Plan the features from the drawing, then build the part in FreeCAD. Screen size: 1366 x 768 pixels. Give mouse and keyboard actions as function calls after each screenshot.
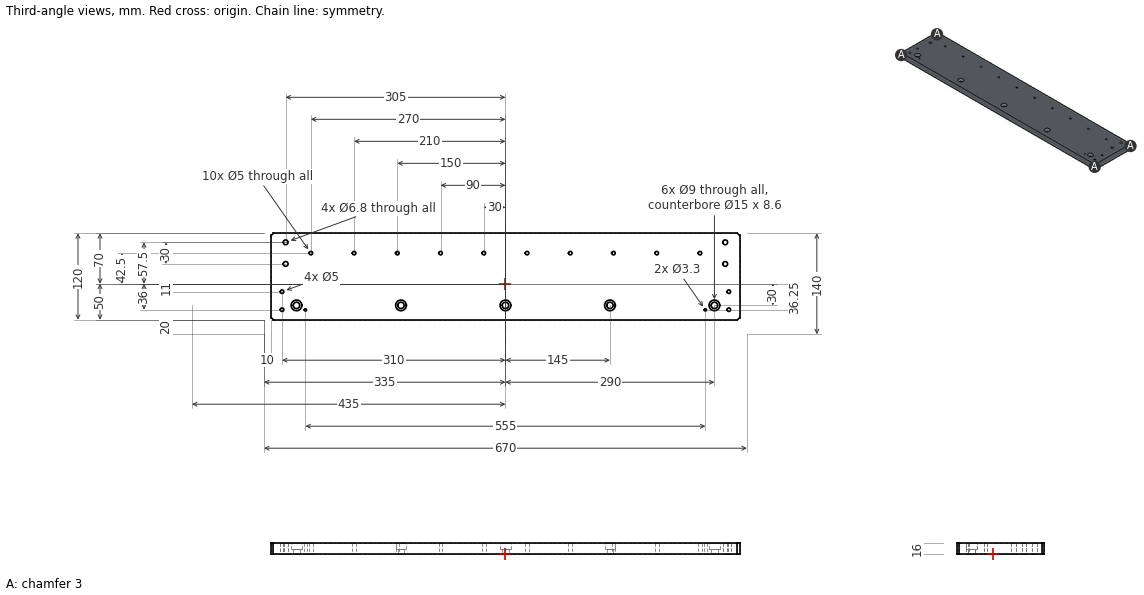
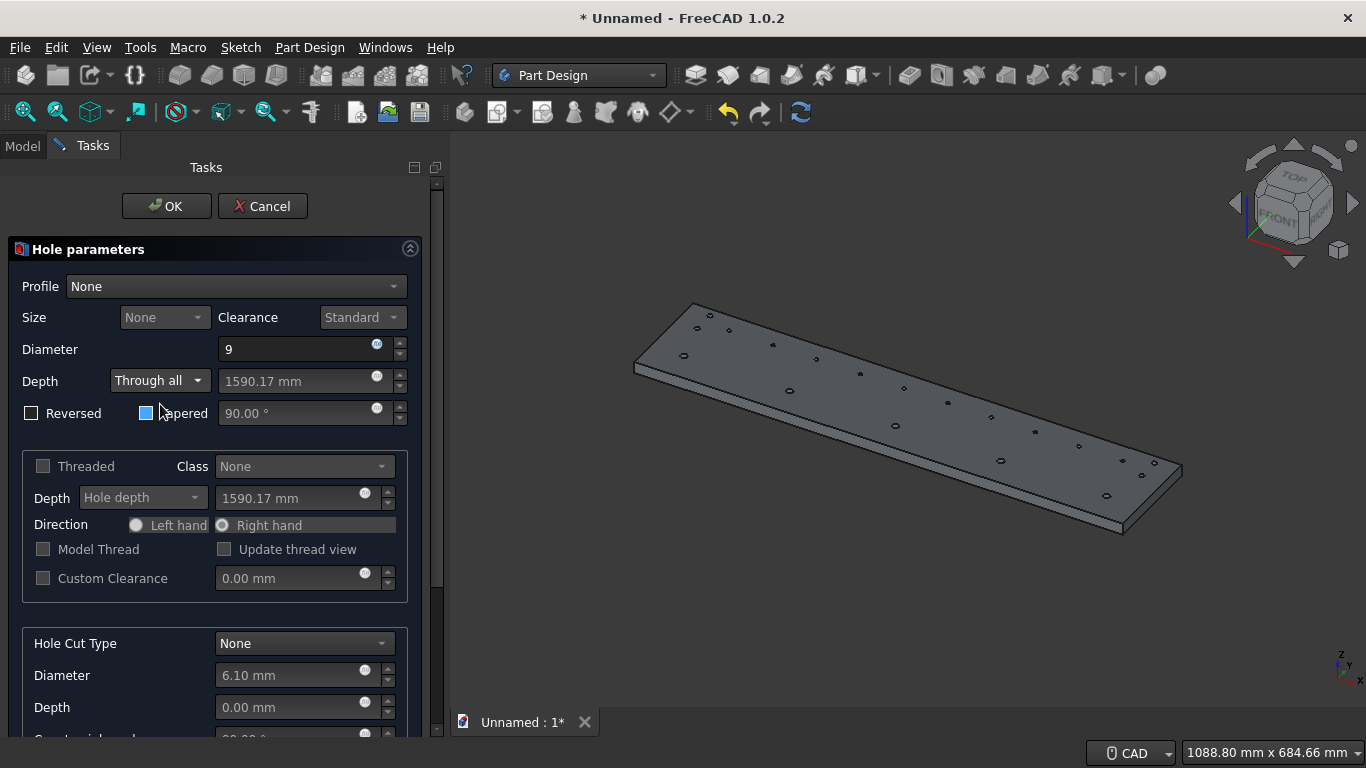
click(306, 644)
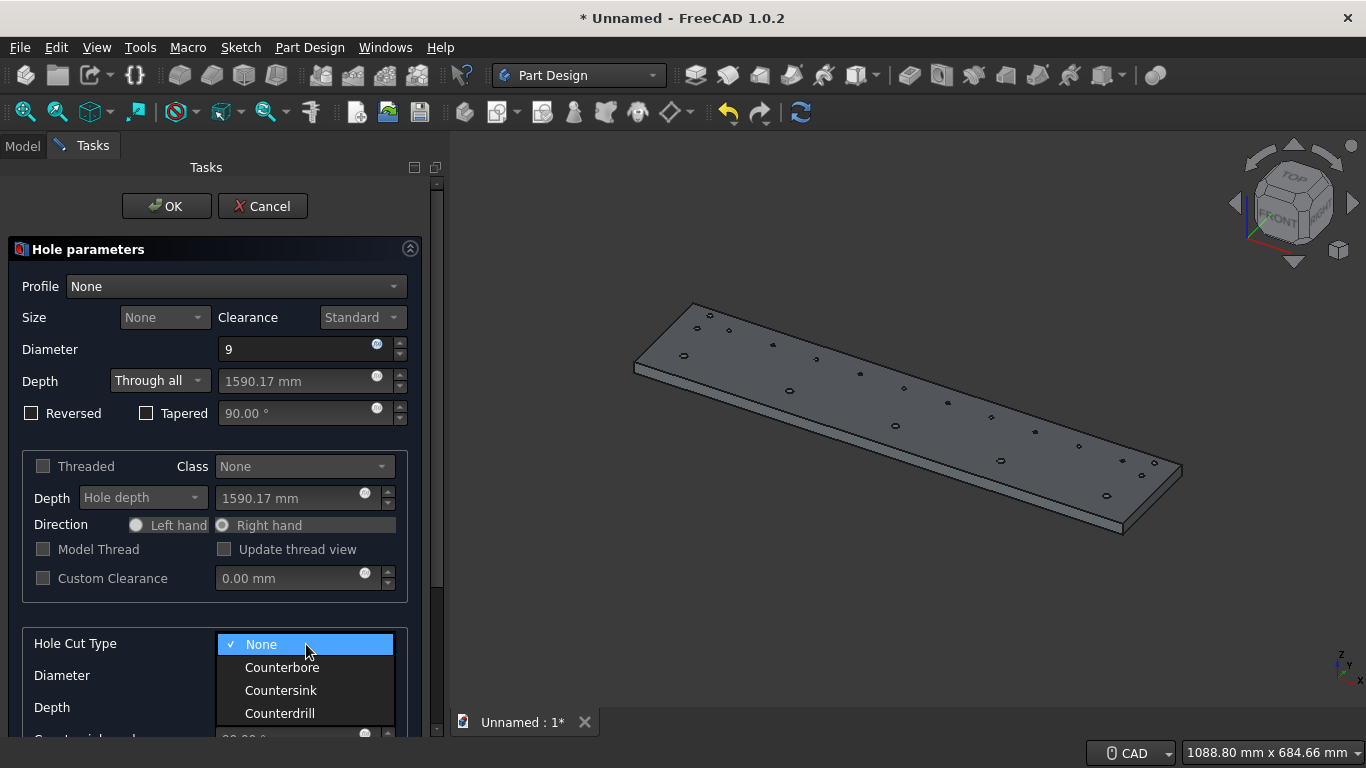
click(304, 668)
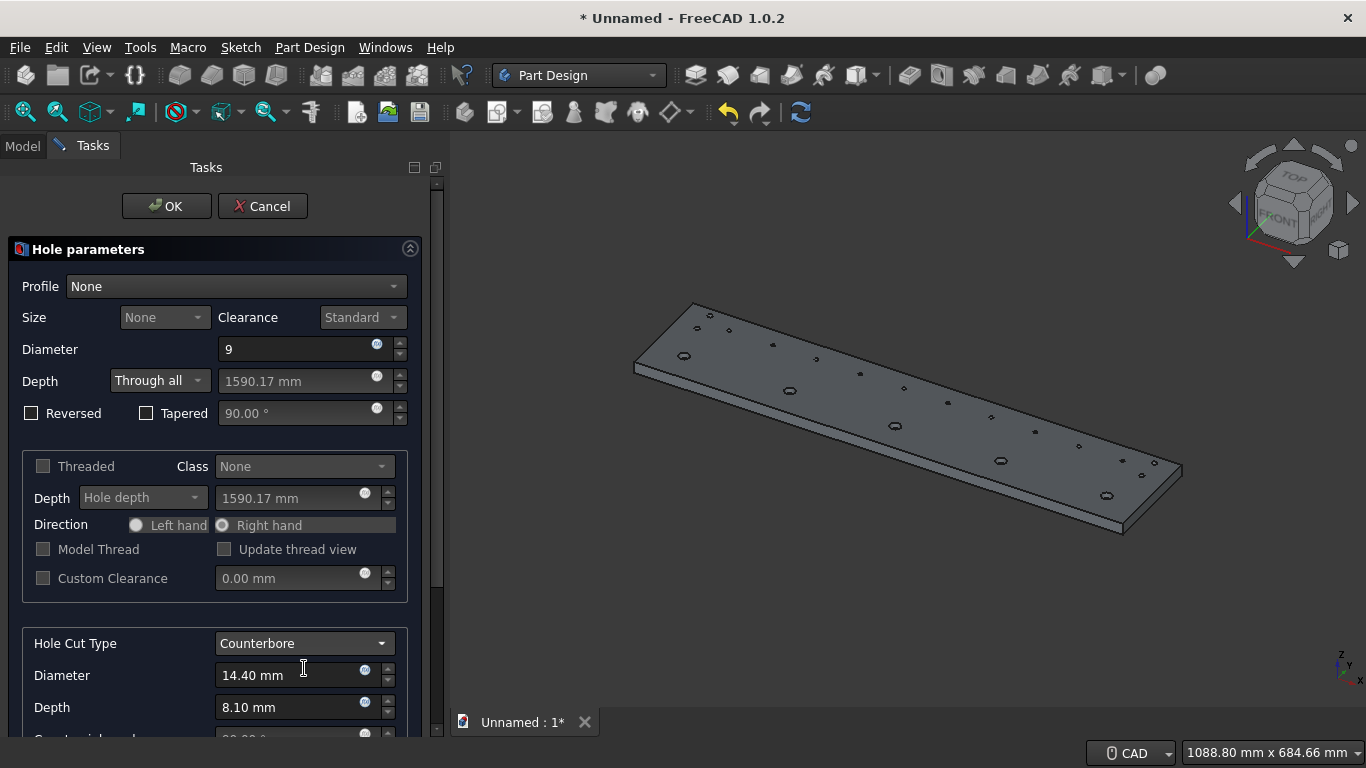
triple_click(298, 675)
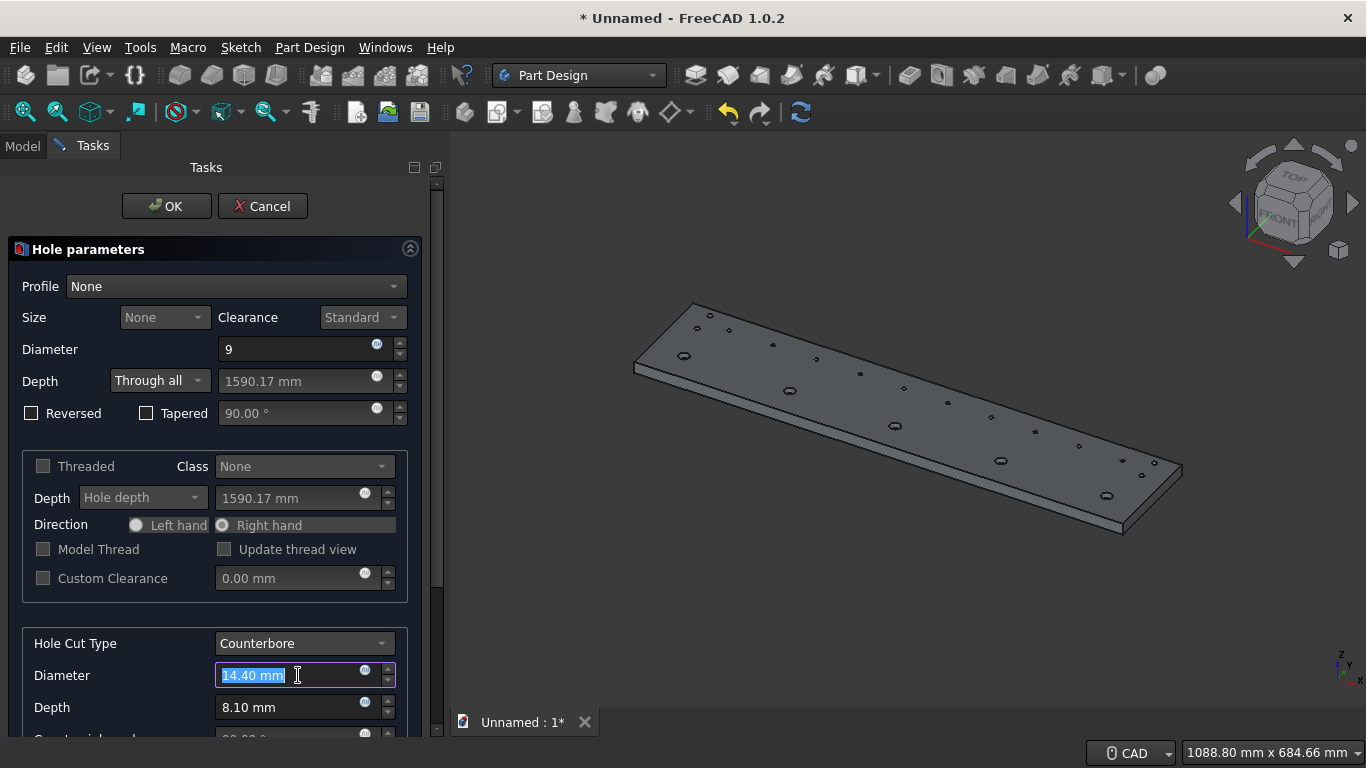
text(15)
key(Tab)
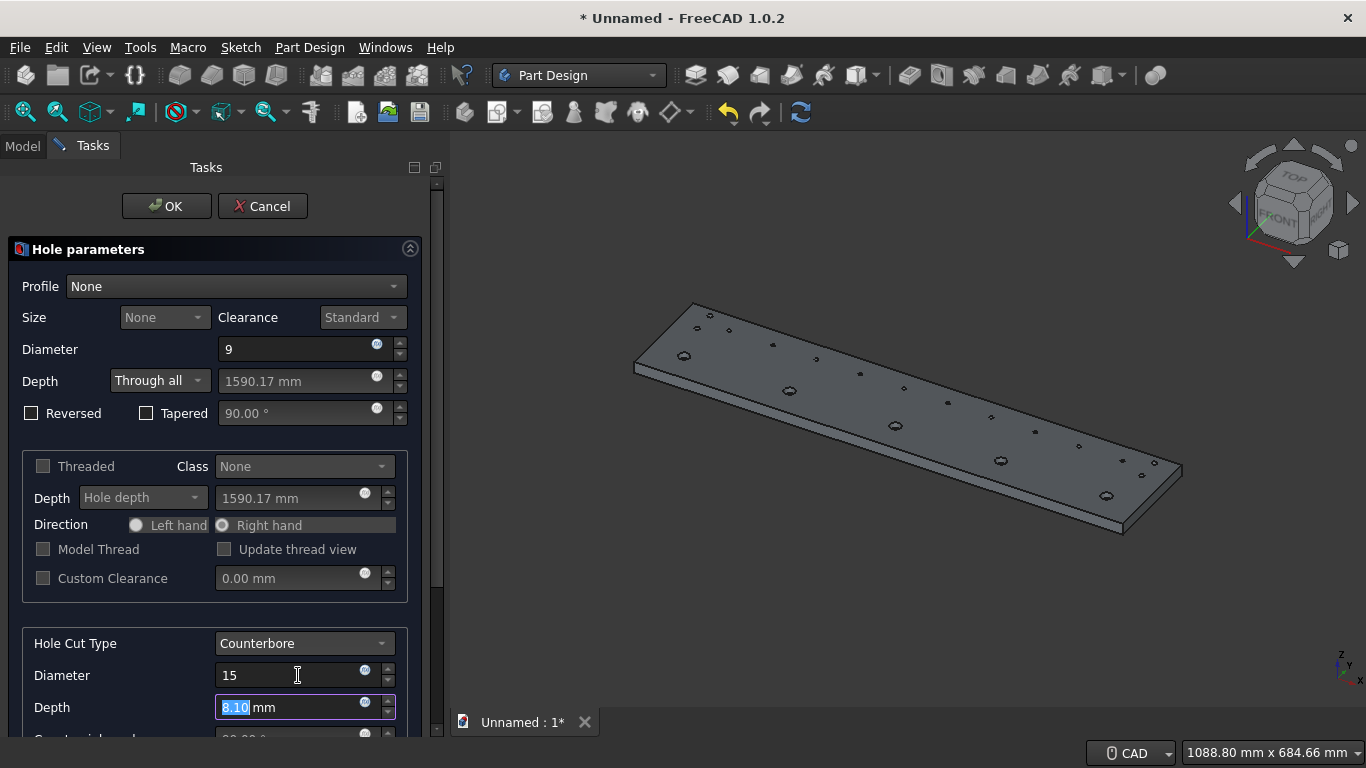
text(8.6)
key(Tab)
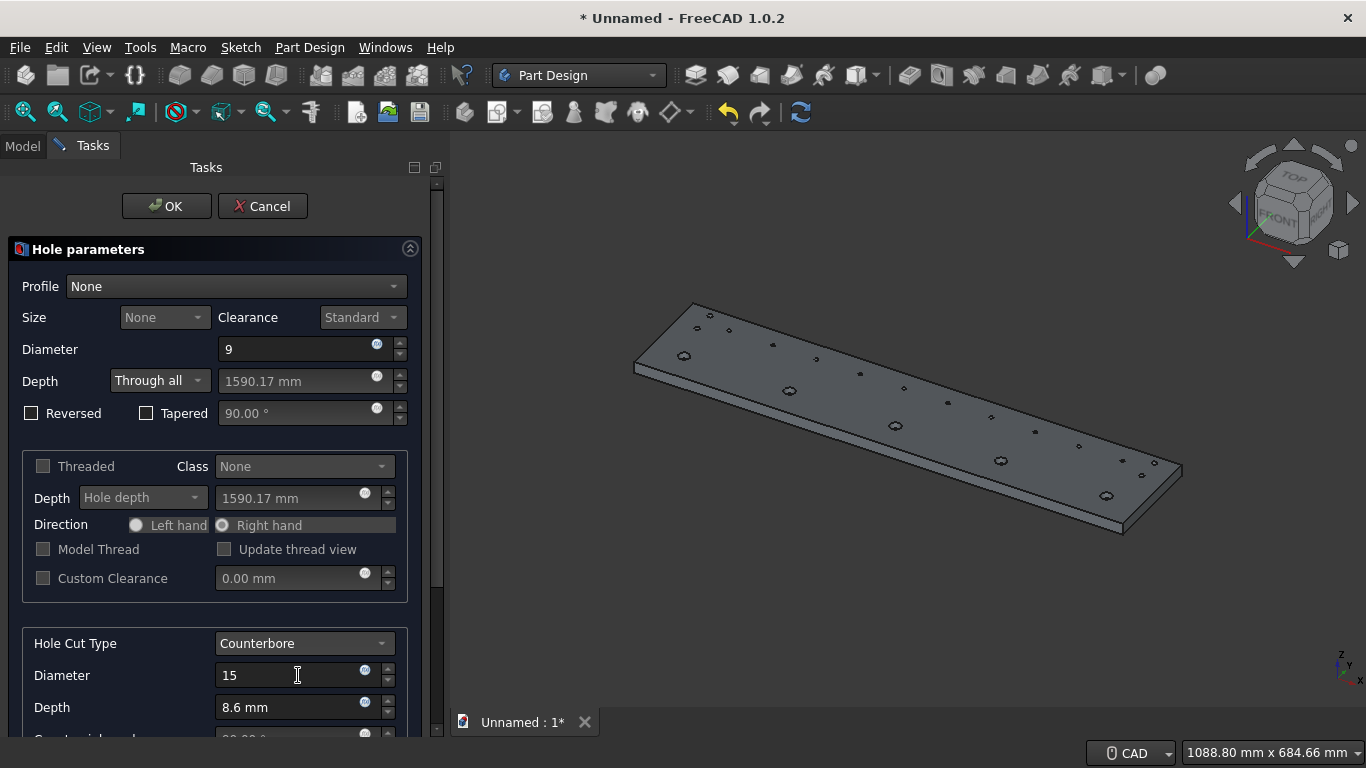
click(167, 206)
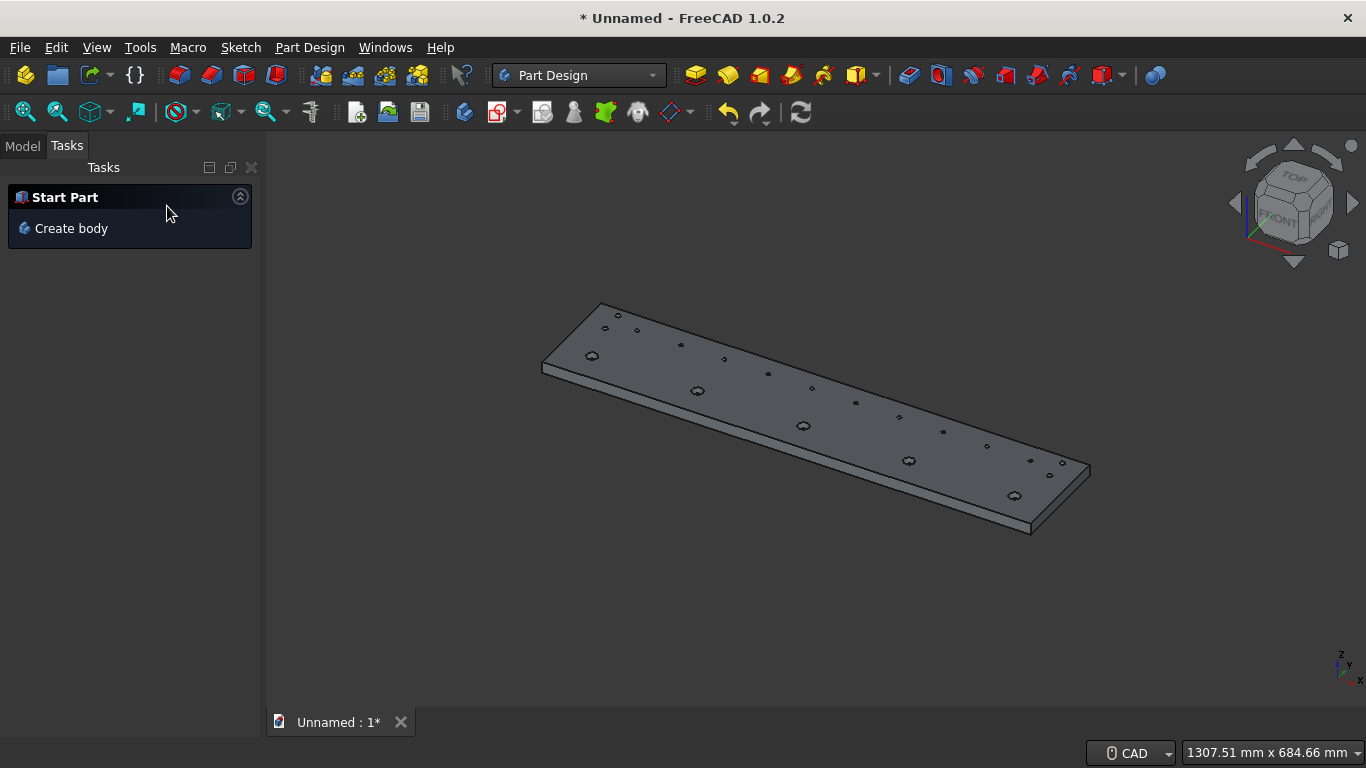
click(677, 366)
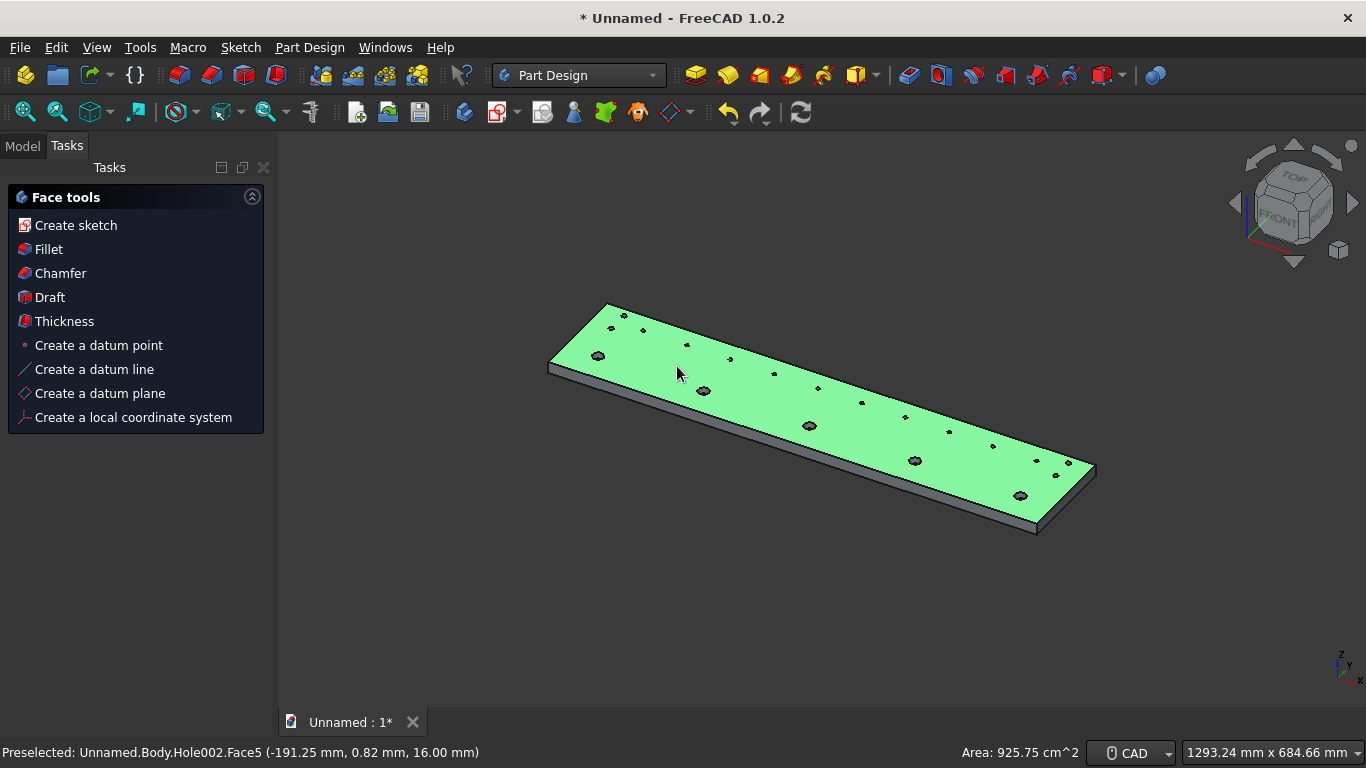
click(498, 112)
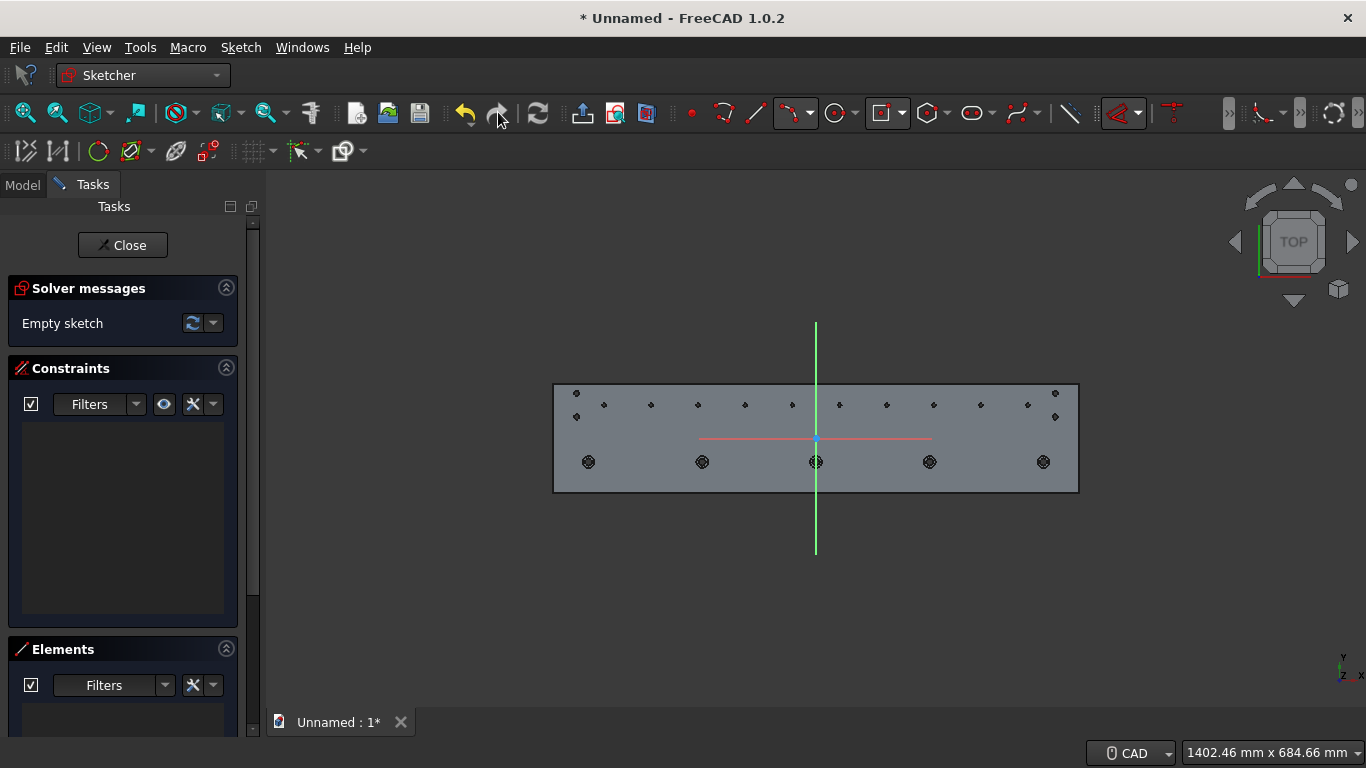
click(904, 114)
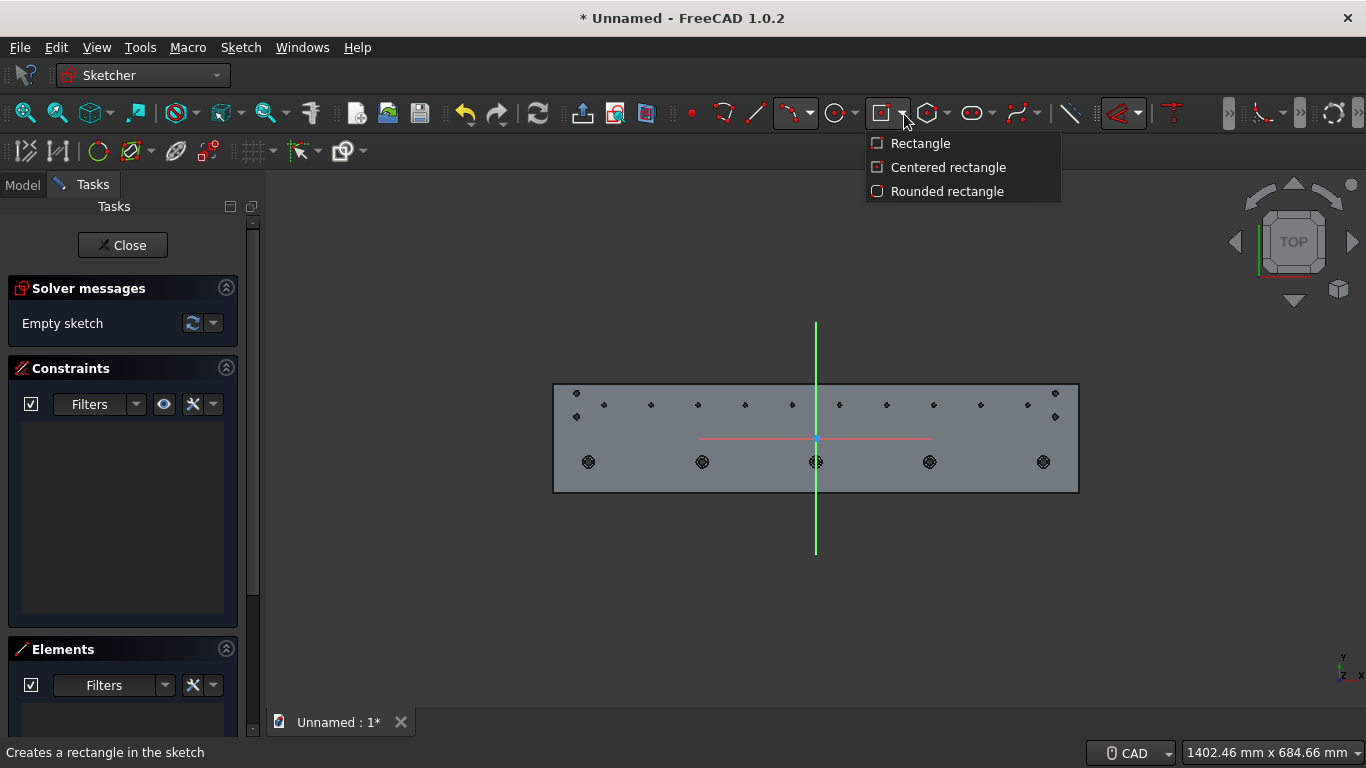
click(964, 143)